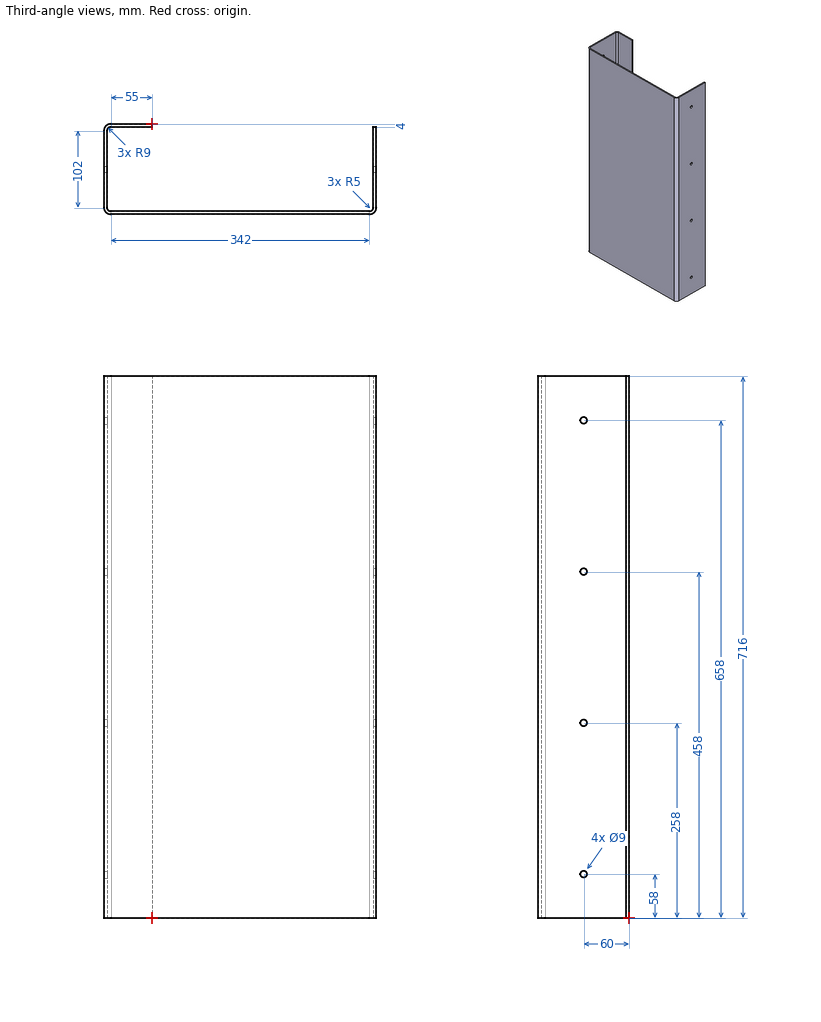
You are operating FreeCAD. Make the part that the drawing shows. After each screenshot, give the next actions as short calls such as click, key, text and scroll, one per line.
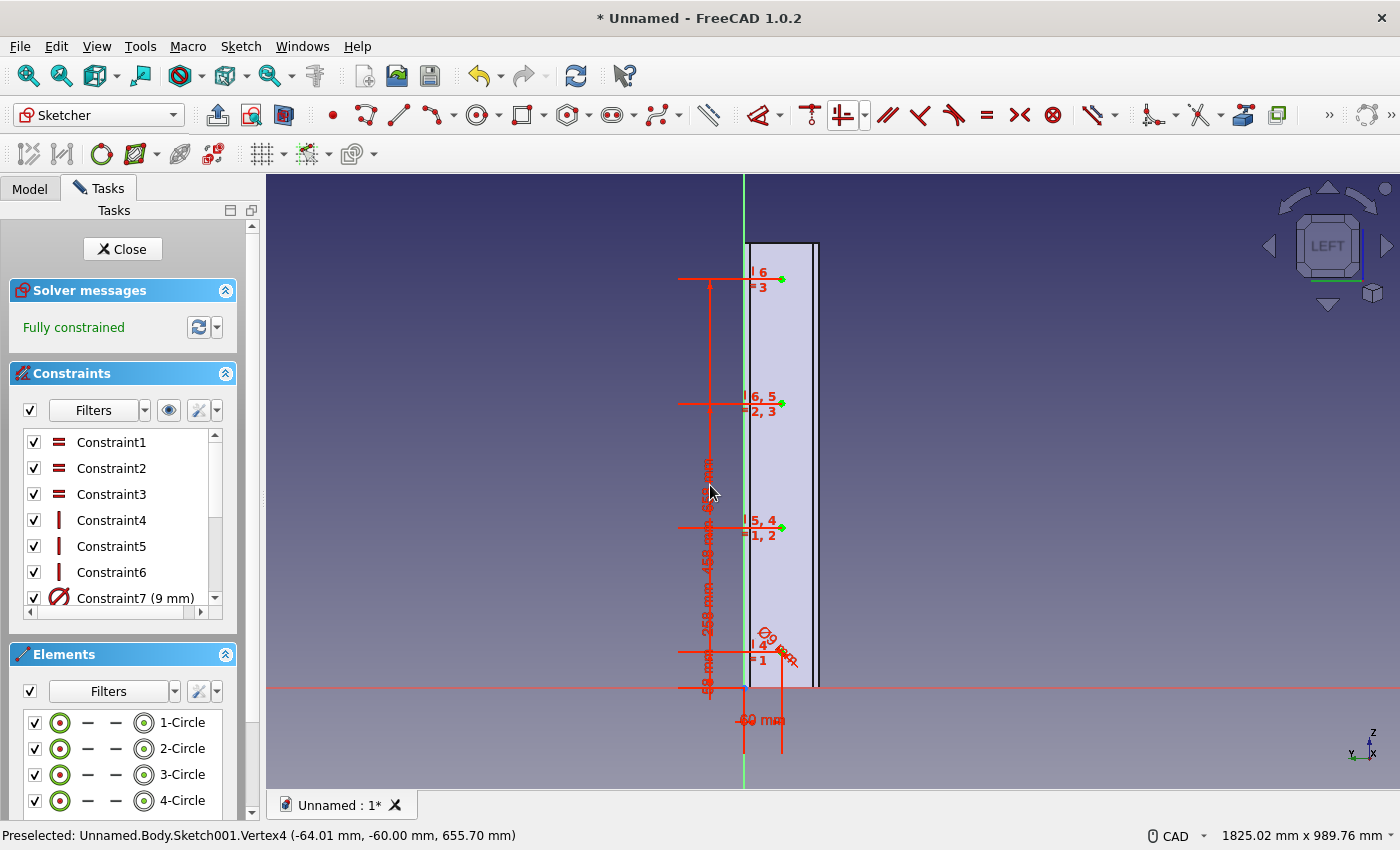
click(123, 249)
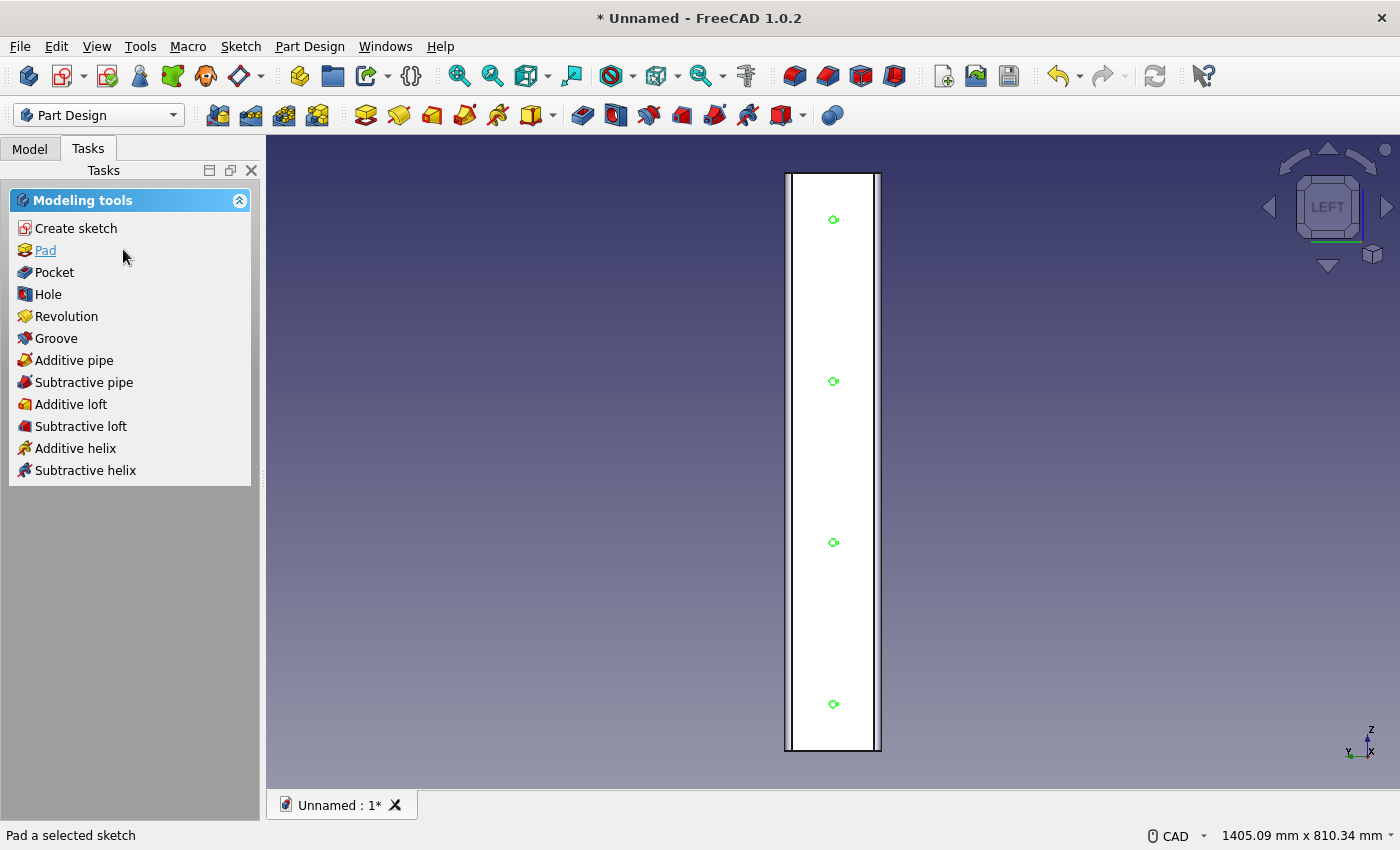
click(583, 116)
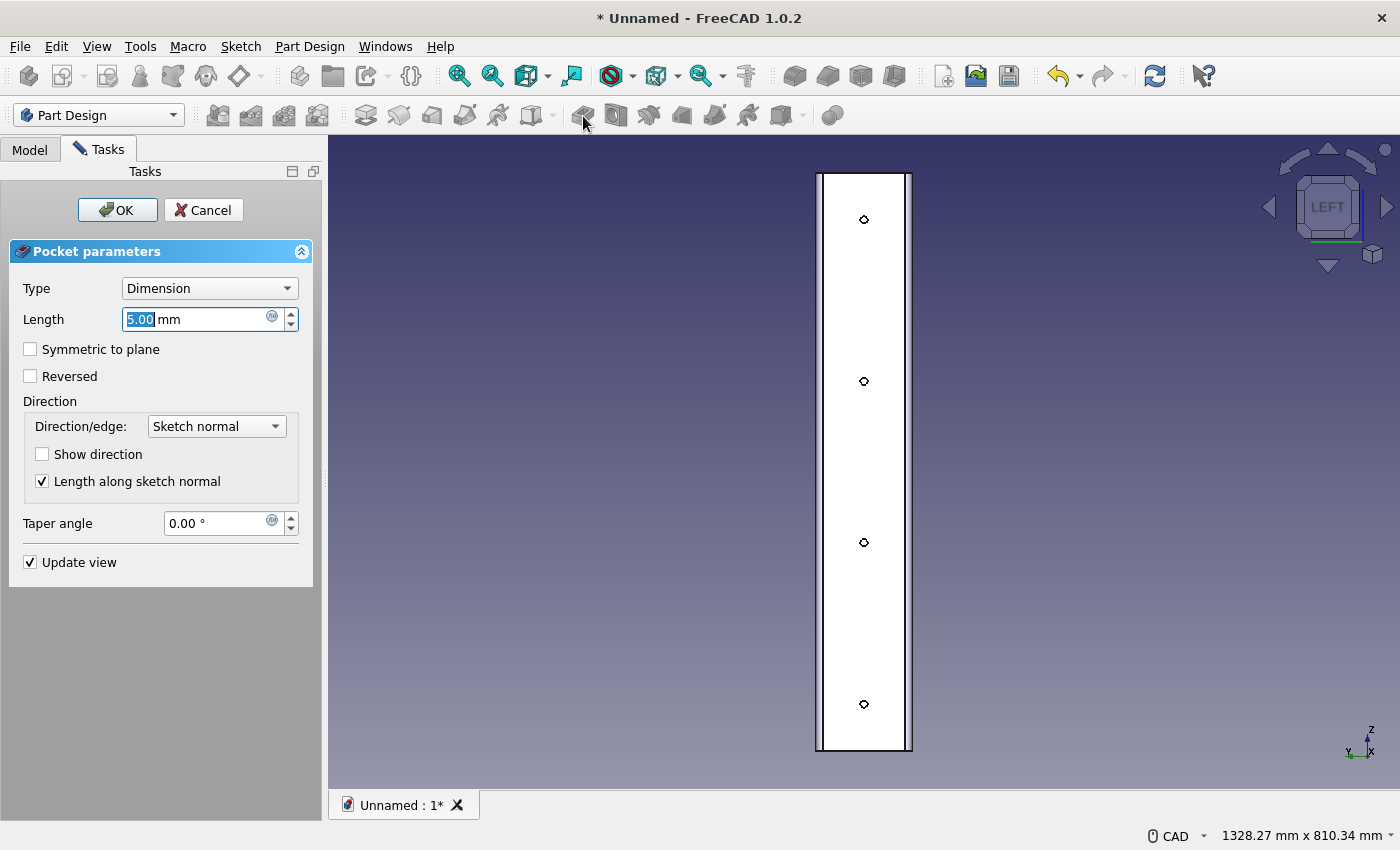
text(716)
key(Tab)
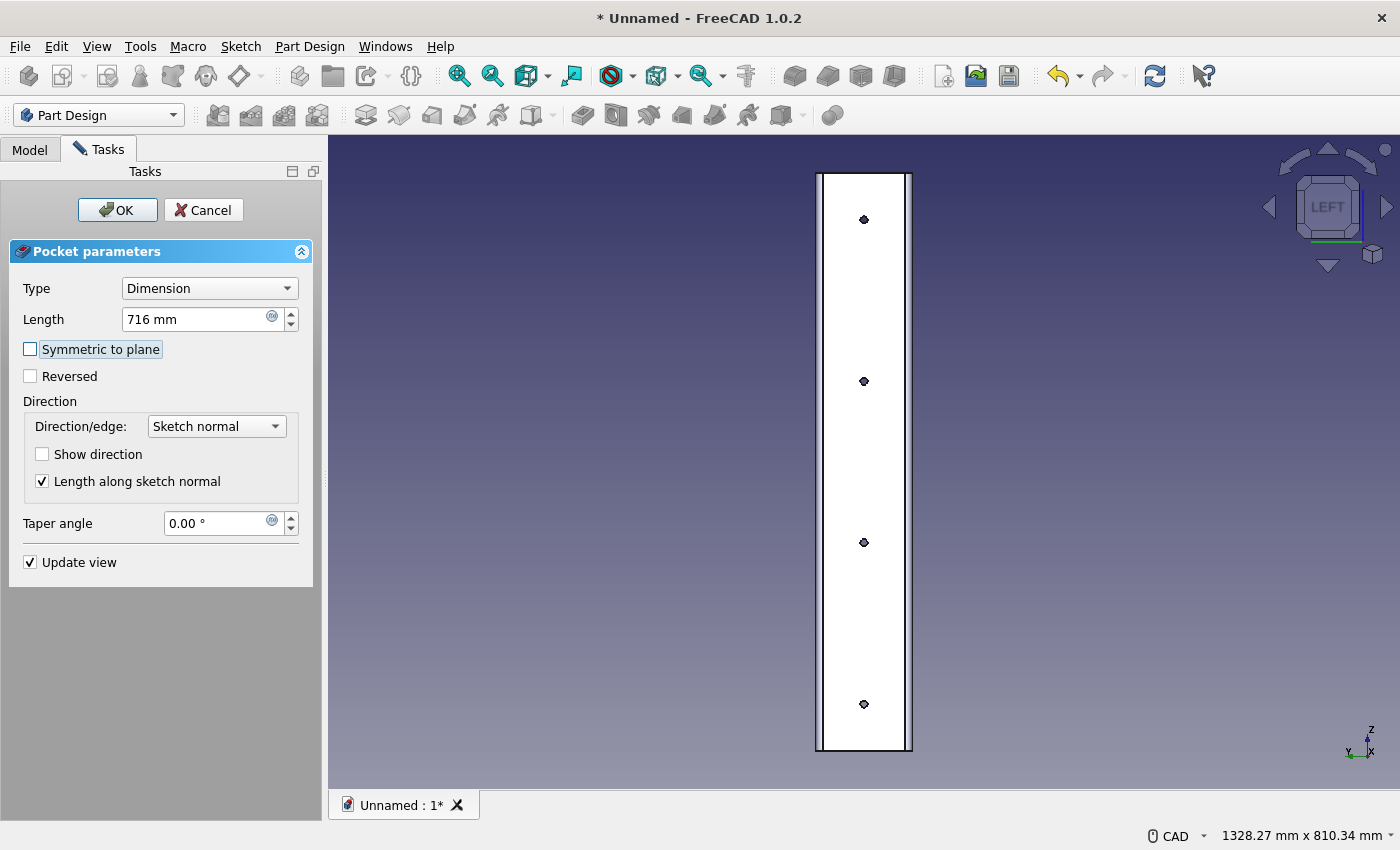
click(118, 210)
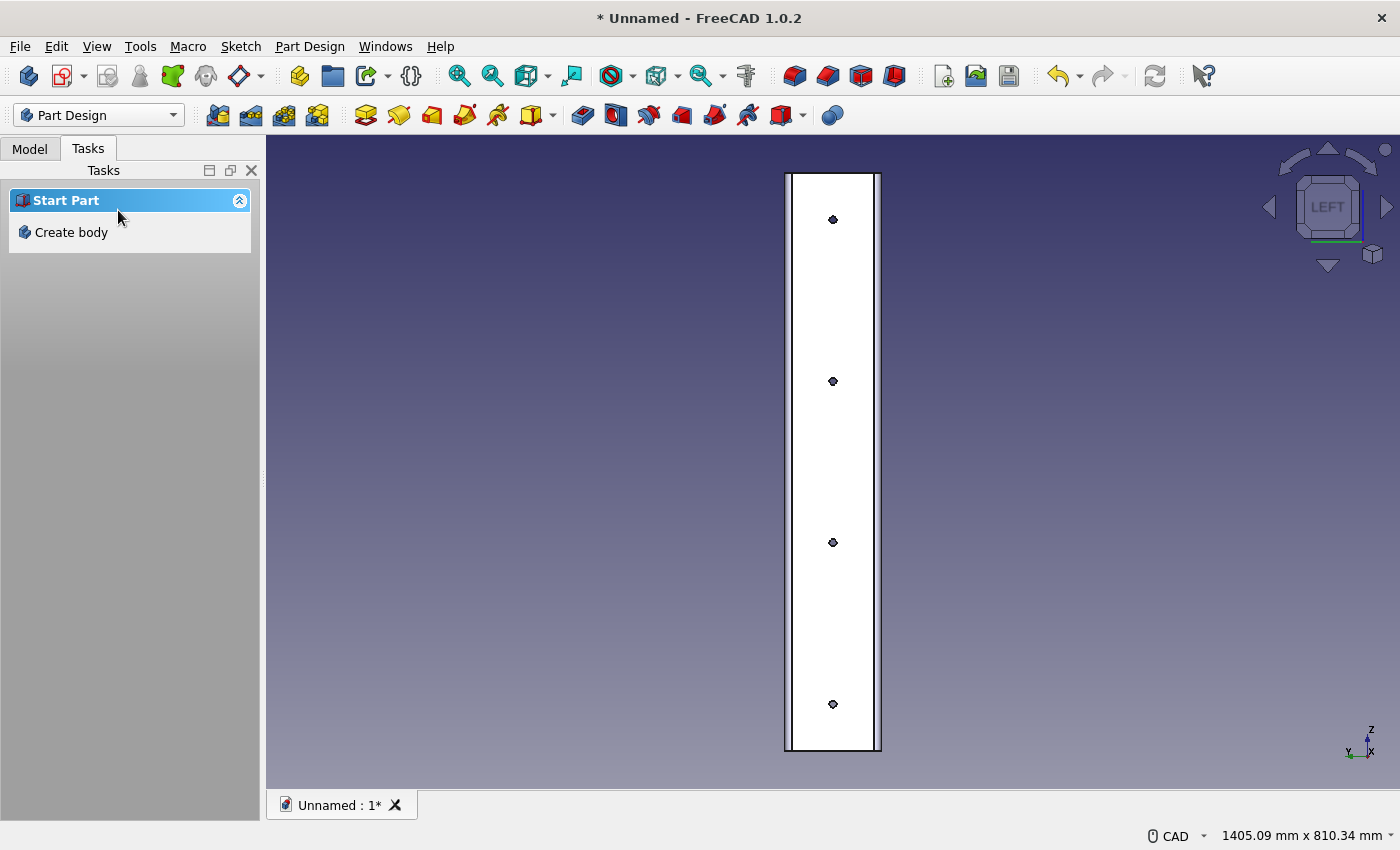
key(0)